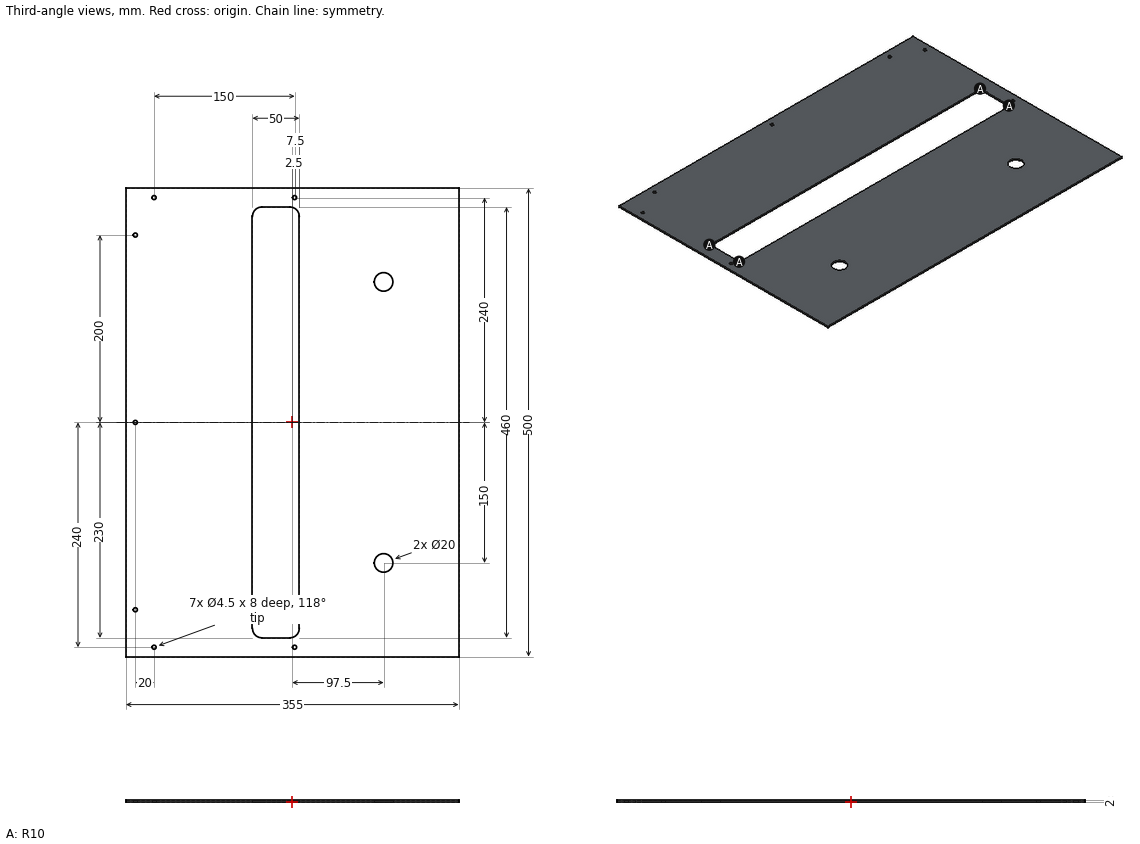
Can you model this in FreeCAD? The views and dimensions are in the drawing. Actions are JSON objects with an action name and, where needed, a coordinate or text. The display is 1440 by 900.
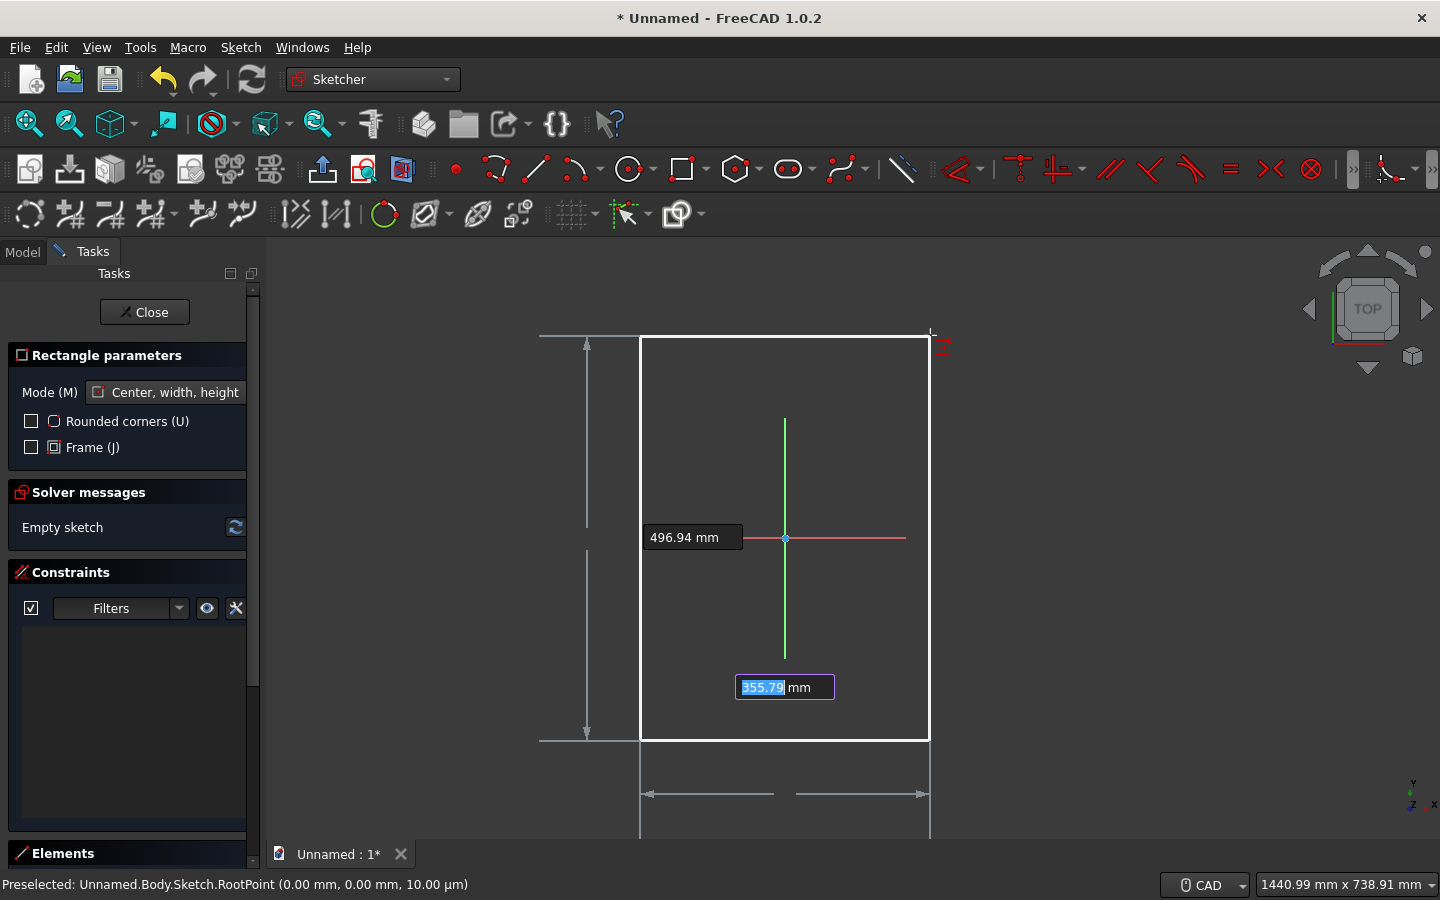
{"action": "type", "text": "355"}
{"action": "key", "text": "Tab"}
{"action": "type", "text": "500"}
{"action": "key", "text": "Return"}
{"action": "key", "text": "Escape"}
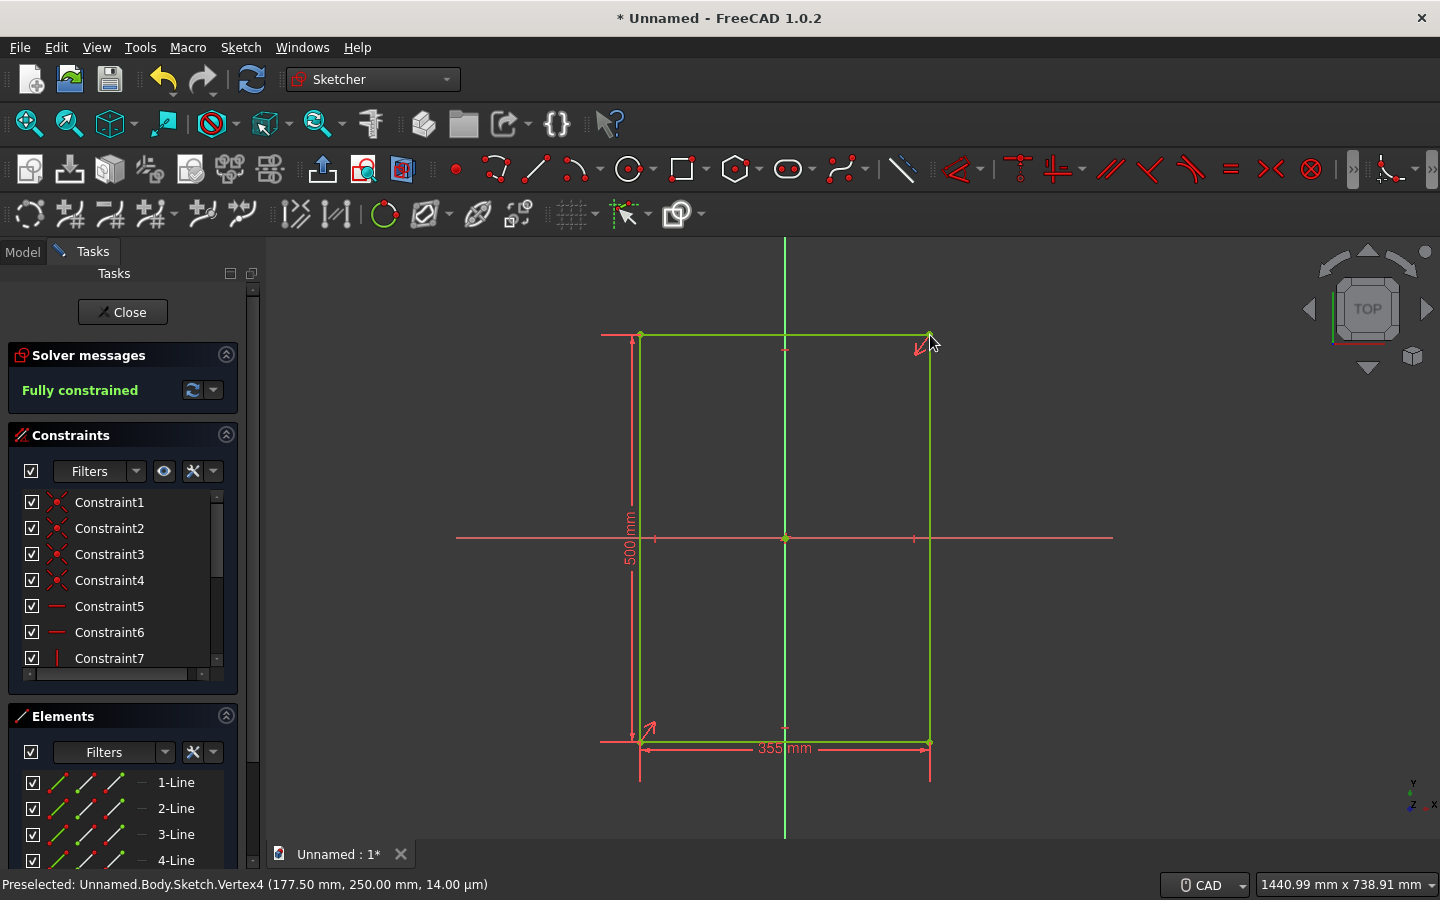
{"action": "left_click", "coordinate": [123, 312]}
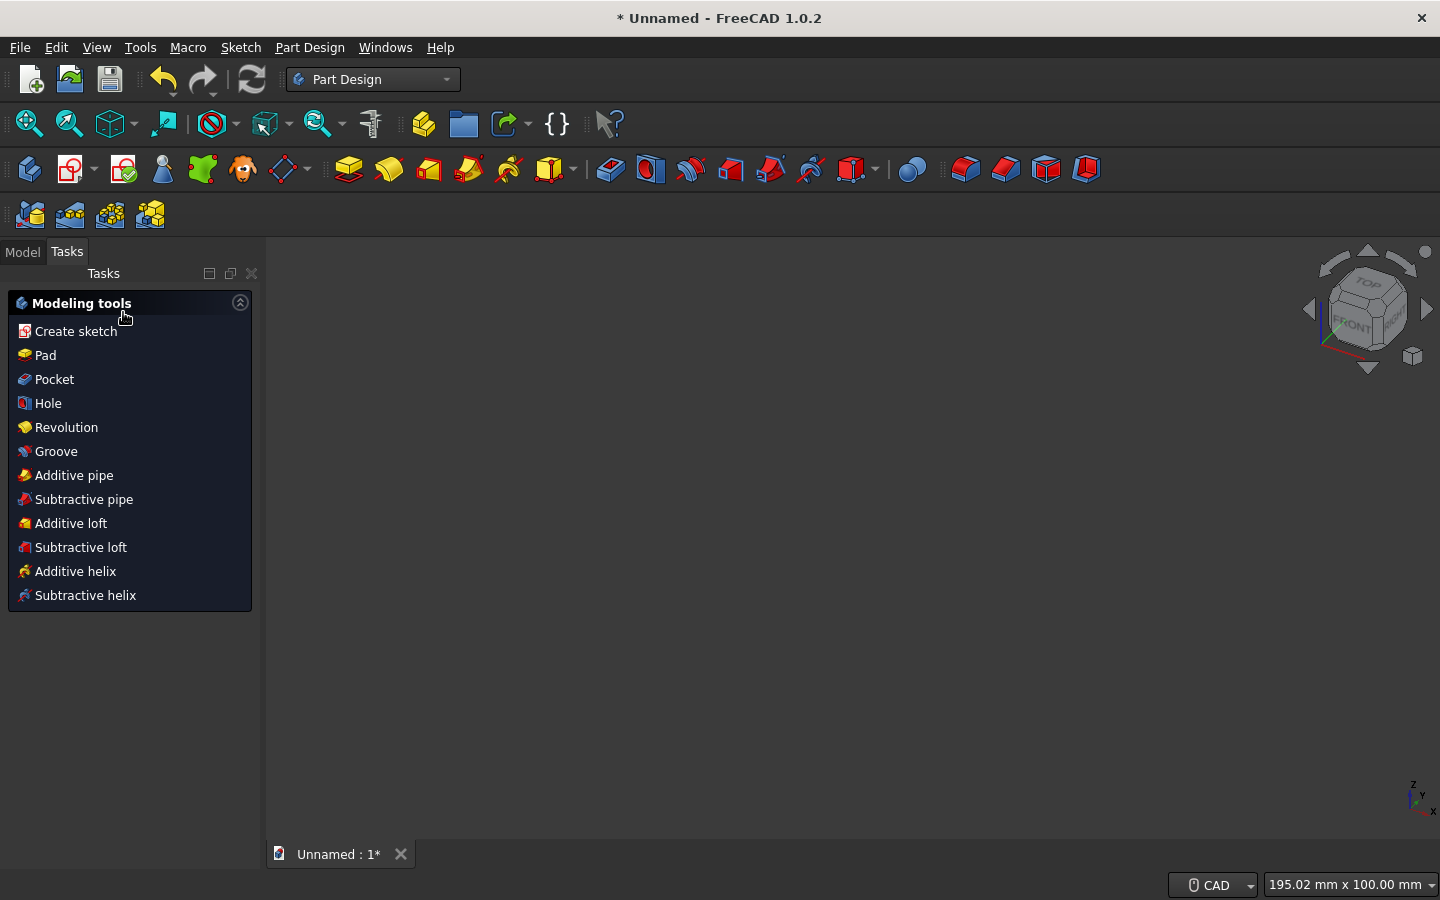
{"action": "left_click", "coordinate": [350, 170]}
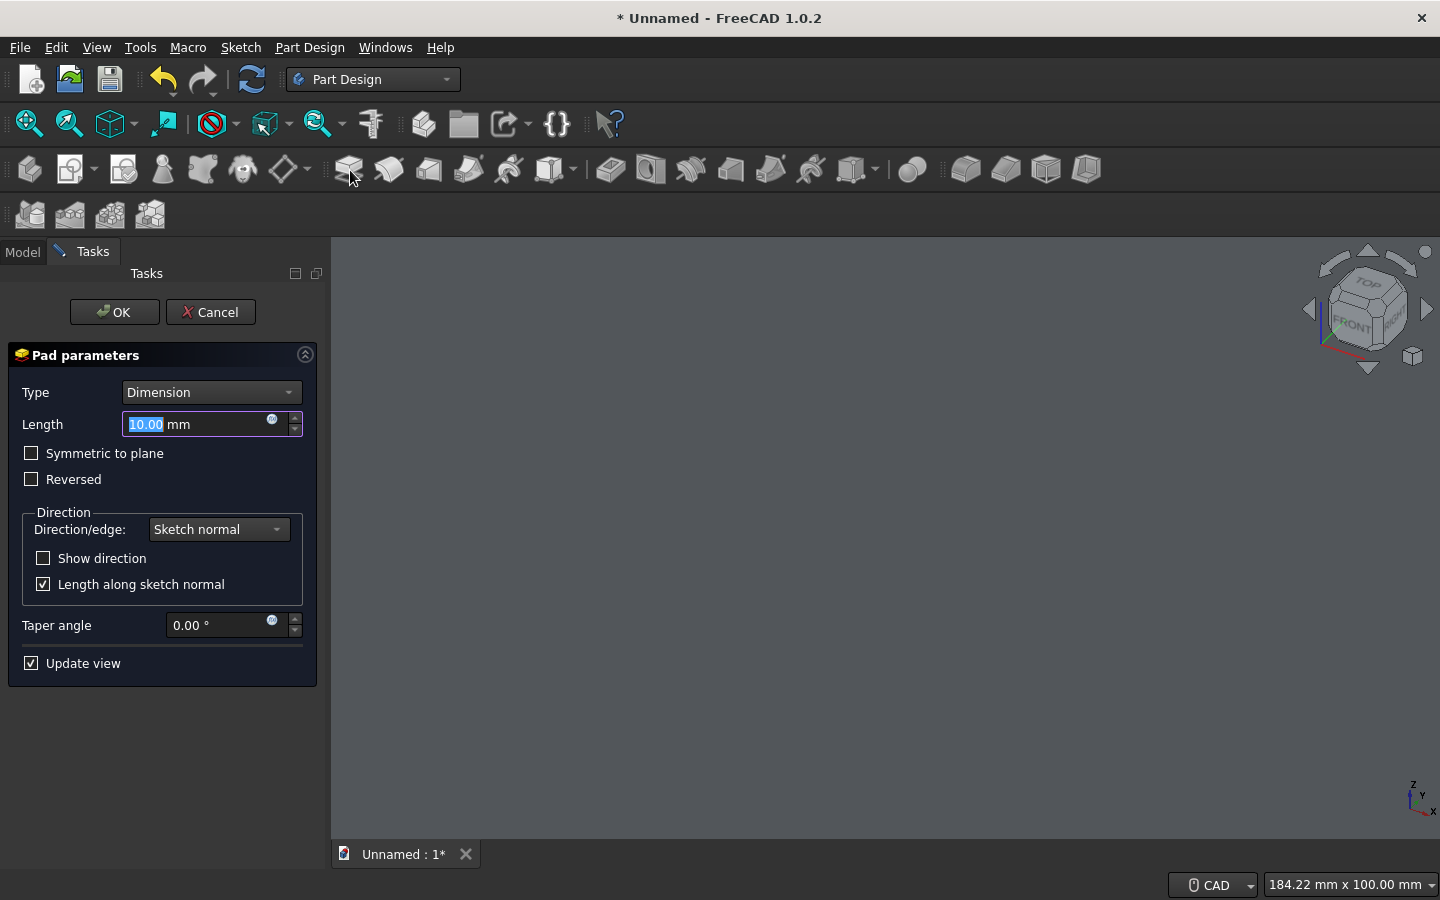
{"action": "type", "text": "2"}
{"action": "key", "text": "Tab"}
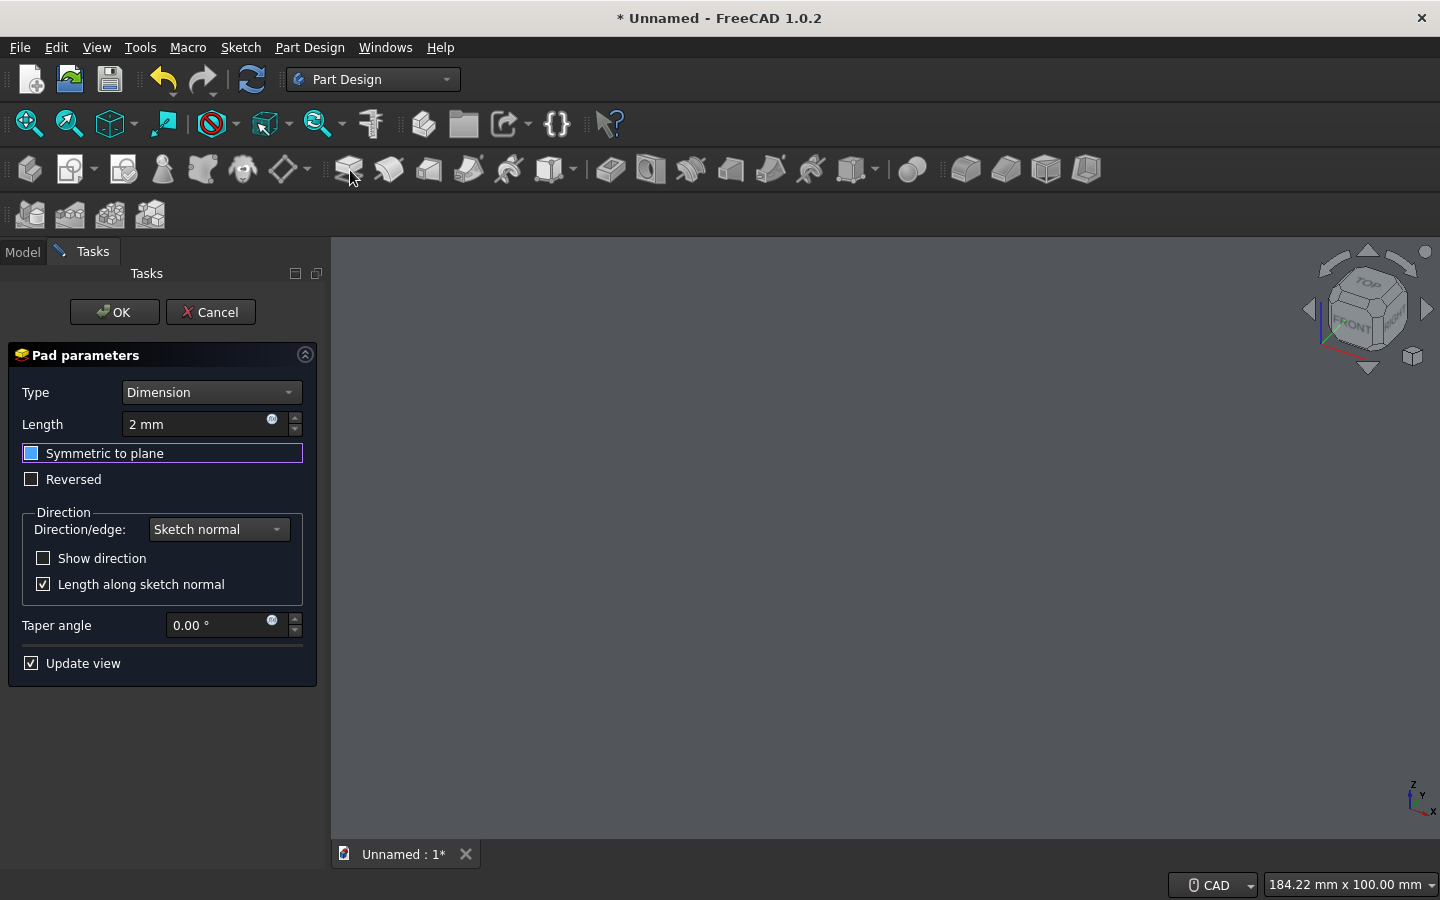
{"action": "left_click", "coordinate": [115, 312]}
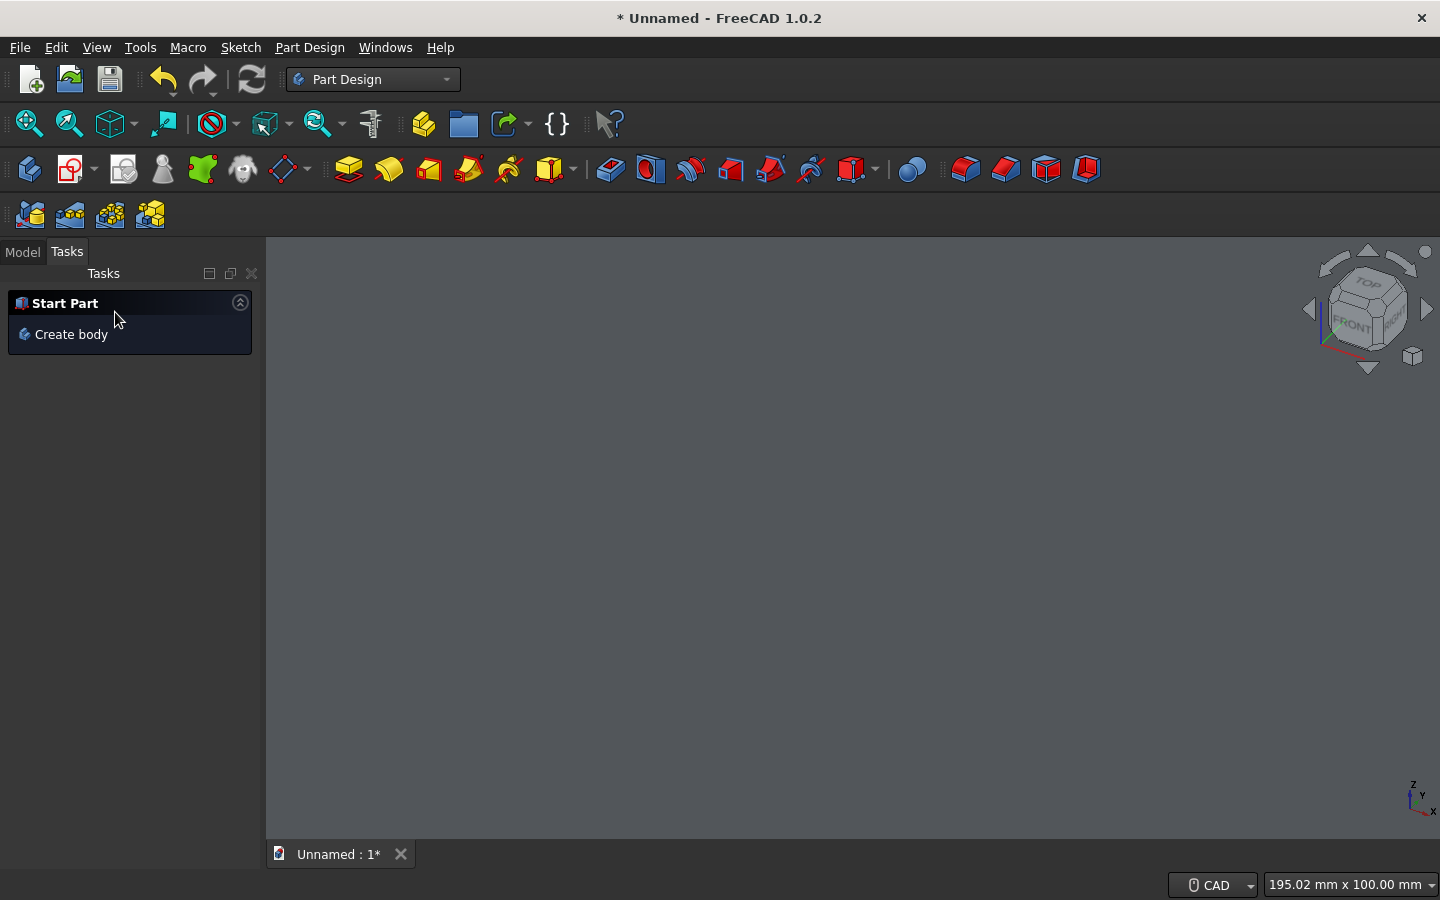
{"action": "left_click", "coordinate": [30, 124]}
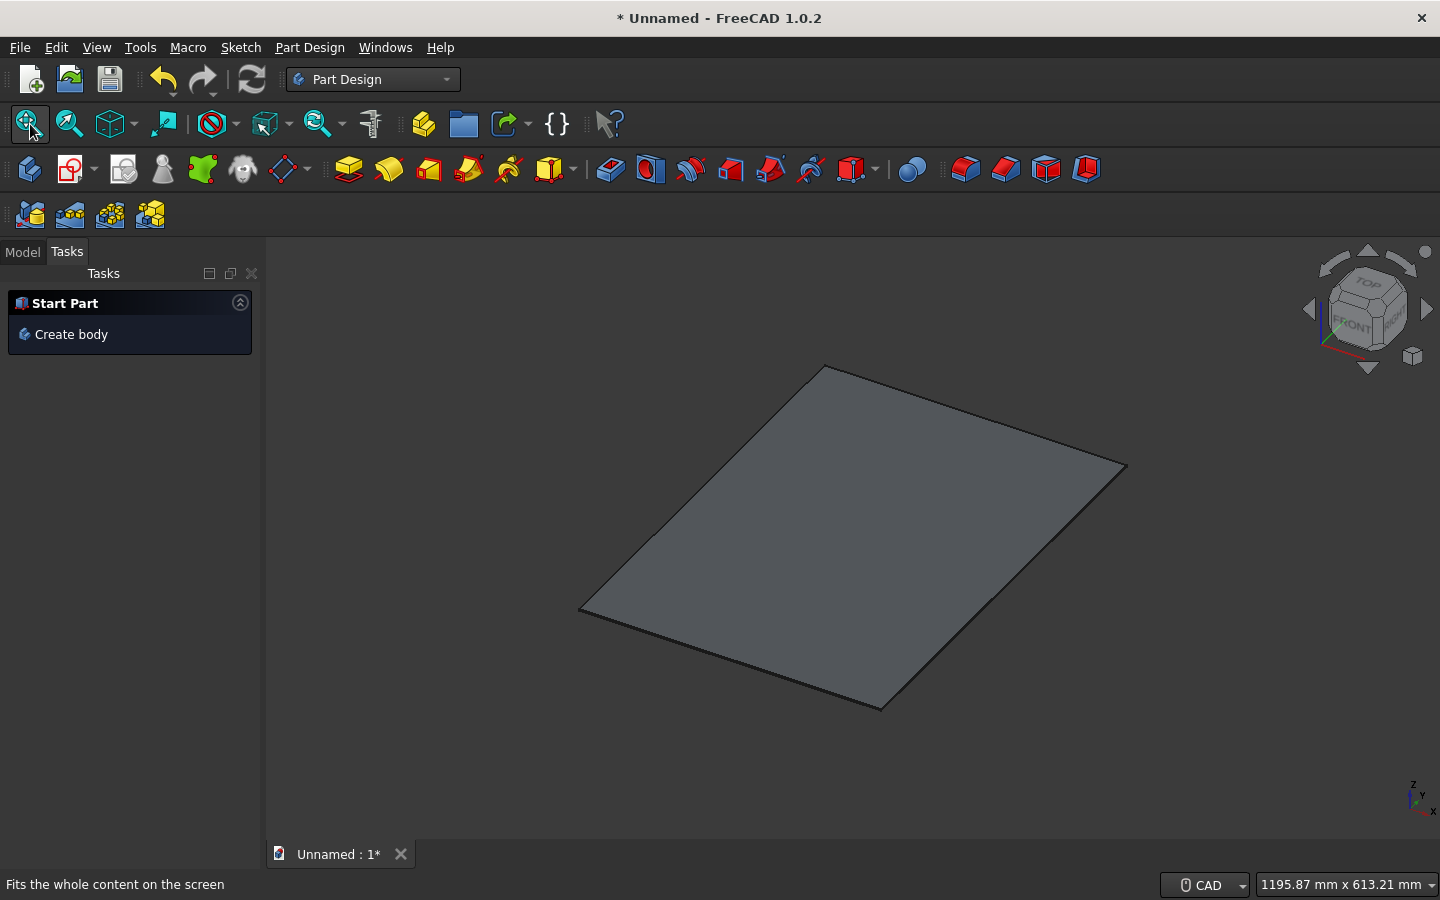
{"action": "left_click", "coordinate": [888, 501]}